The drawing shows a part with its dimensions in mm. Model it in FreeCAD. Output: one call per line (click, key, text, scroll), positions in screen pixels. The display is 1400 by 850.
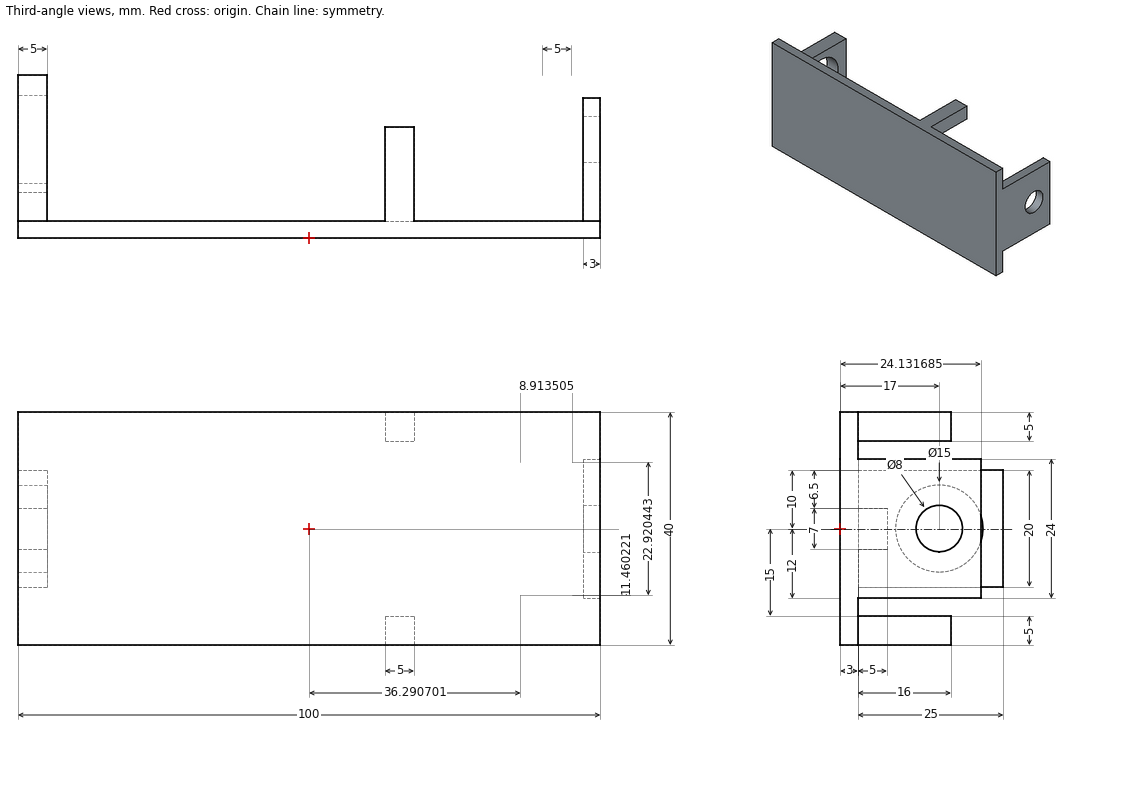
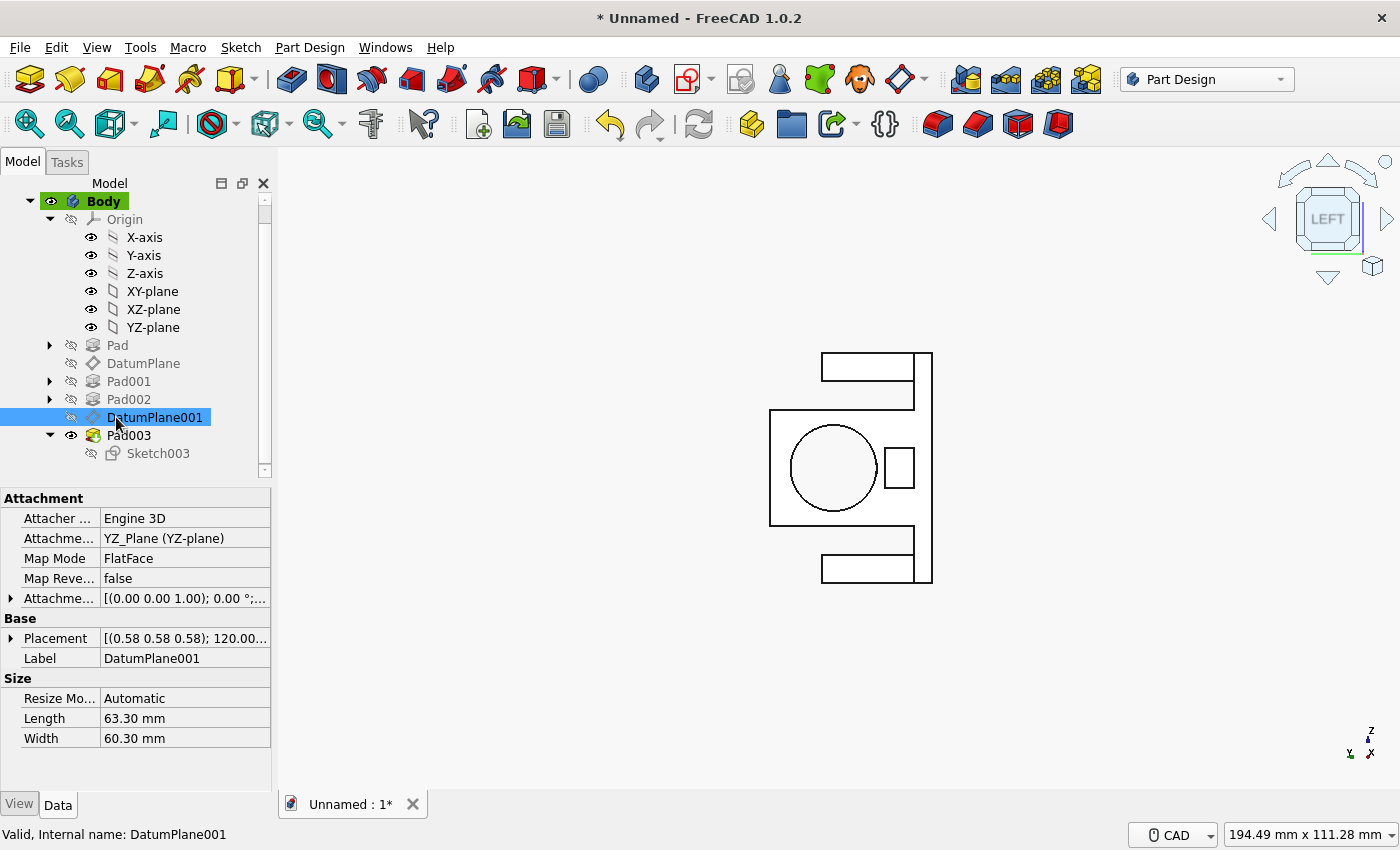
key(v)
key(f)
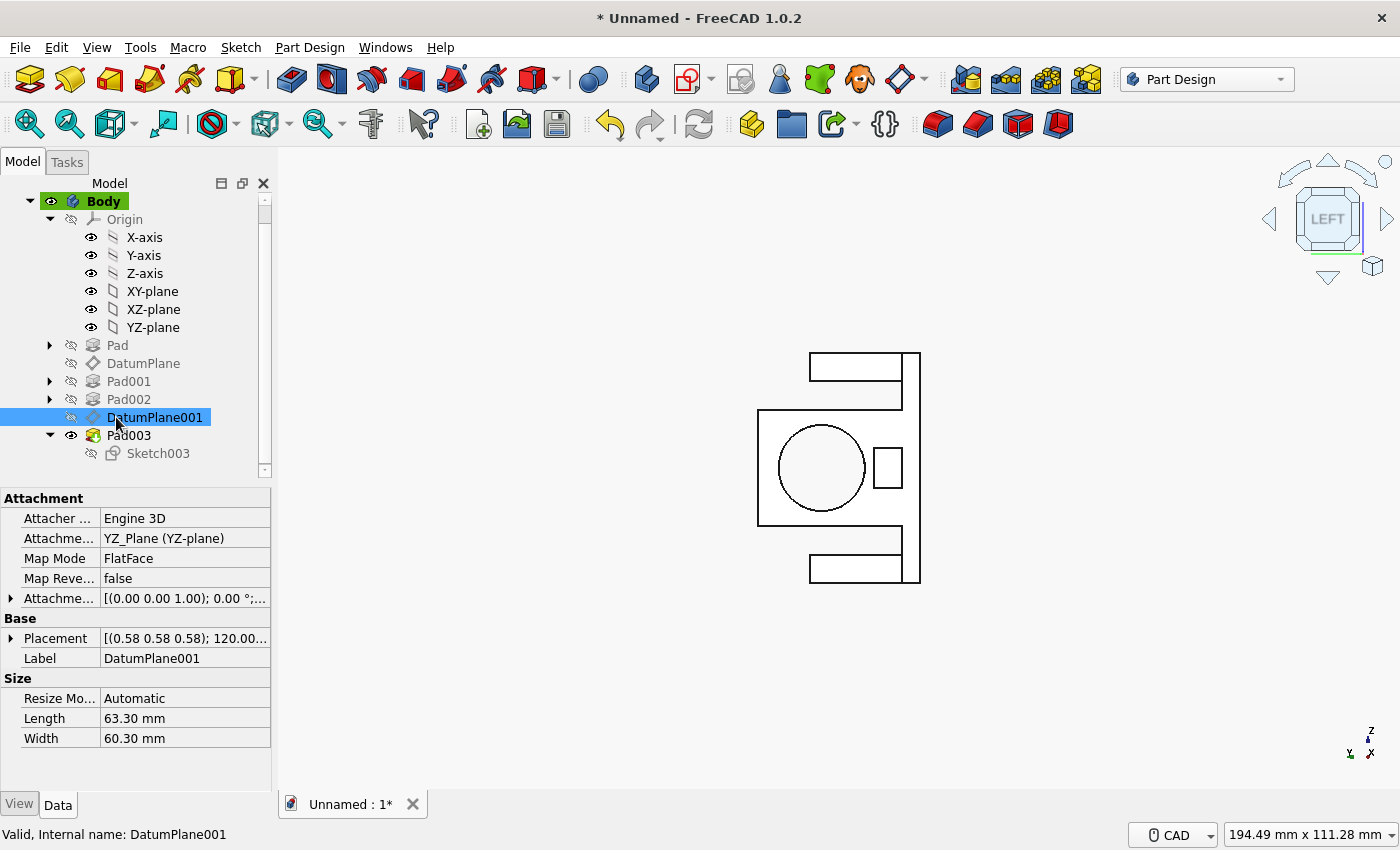
key(0)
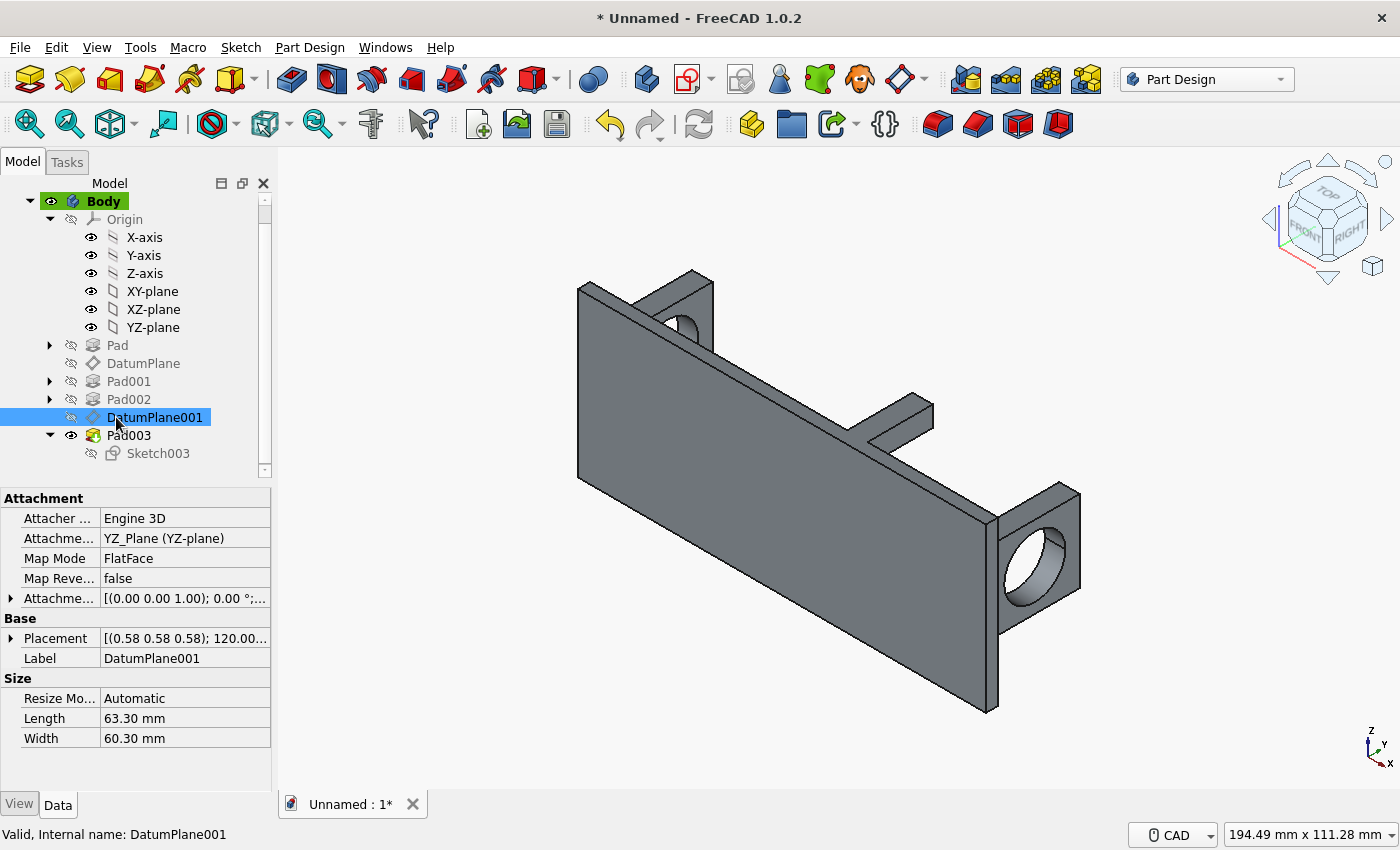
click(994, 532)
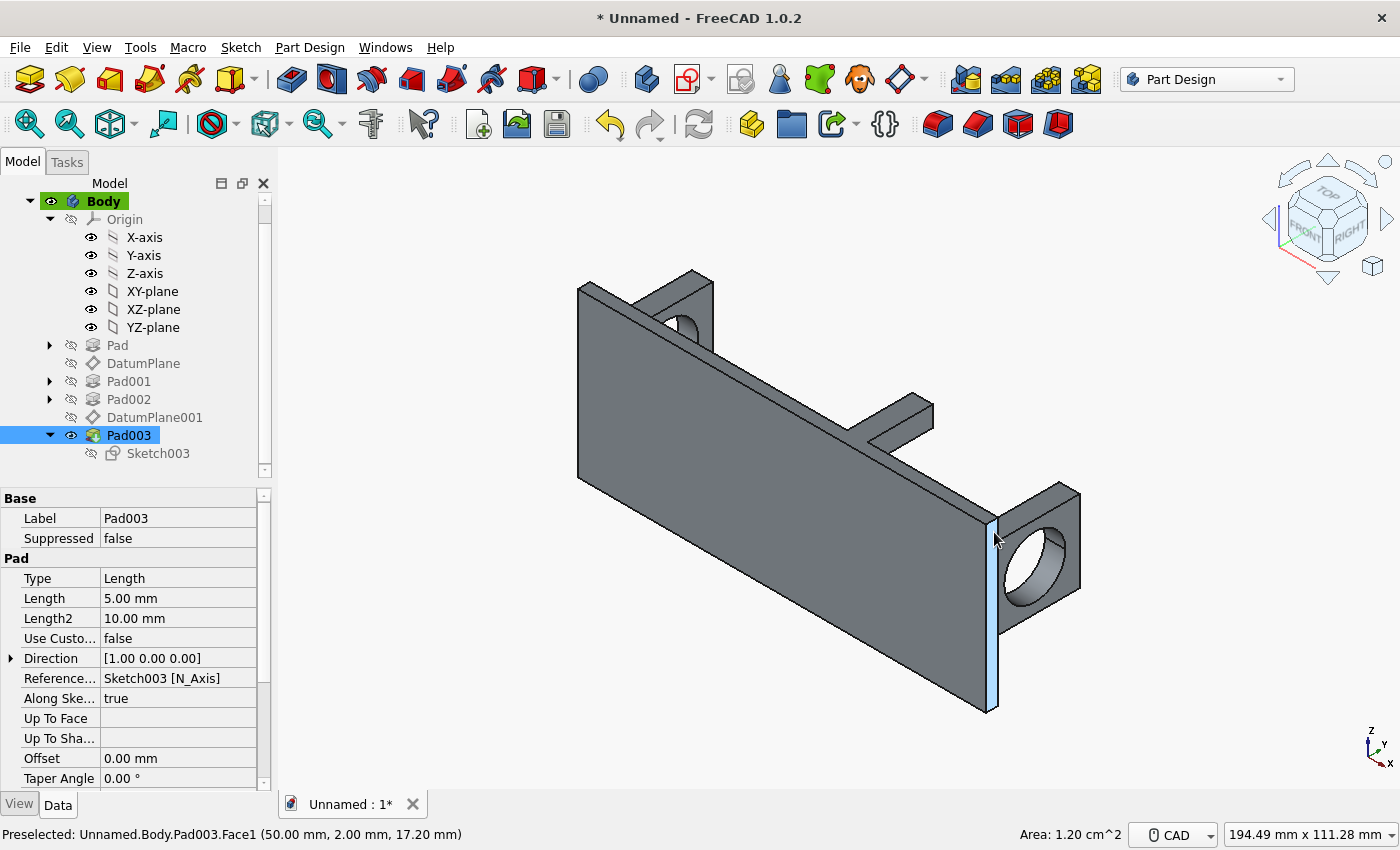
click(688, 80)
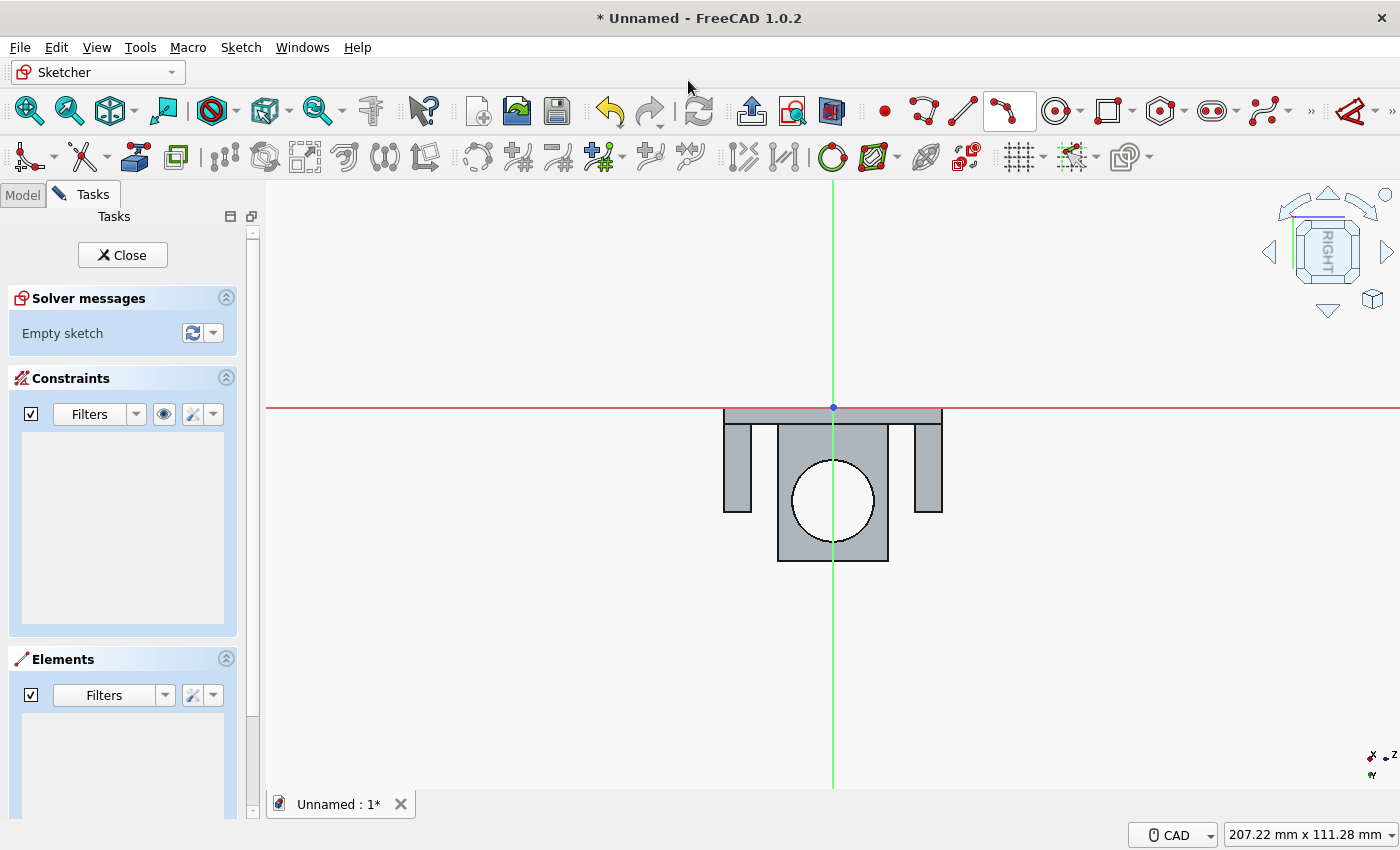
scroll(873, 468, up, 5)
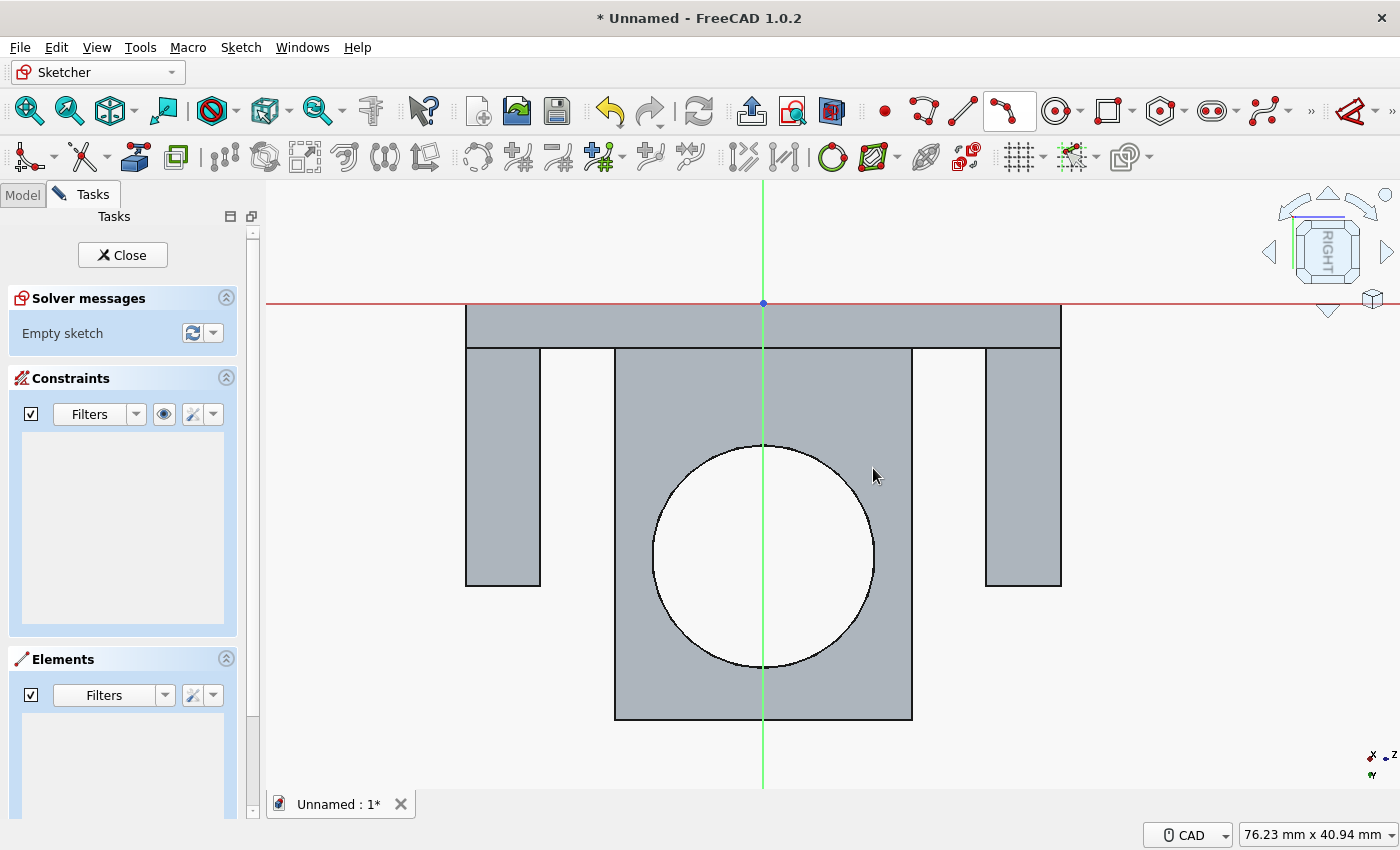
click(1108, 112)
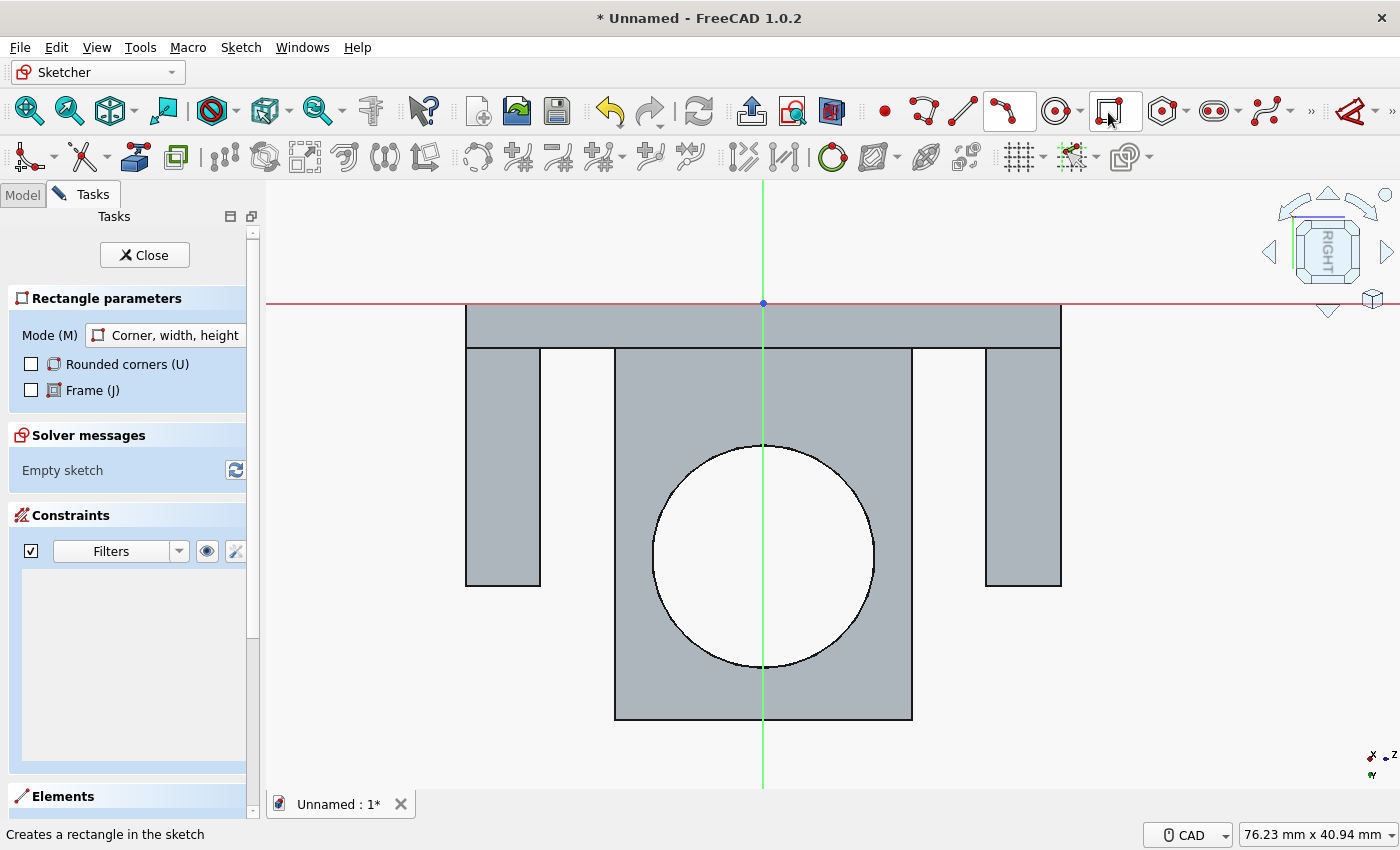
click(585, 304)
move(942, 663)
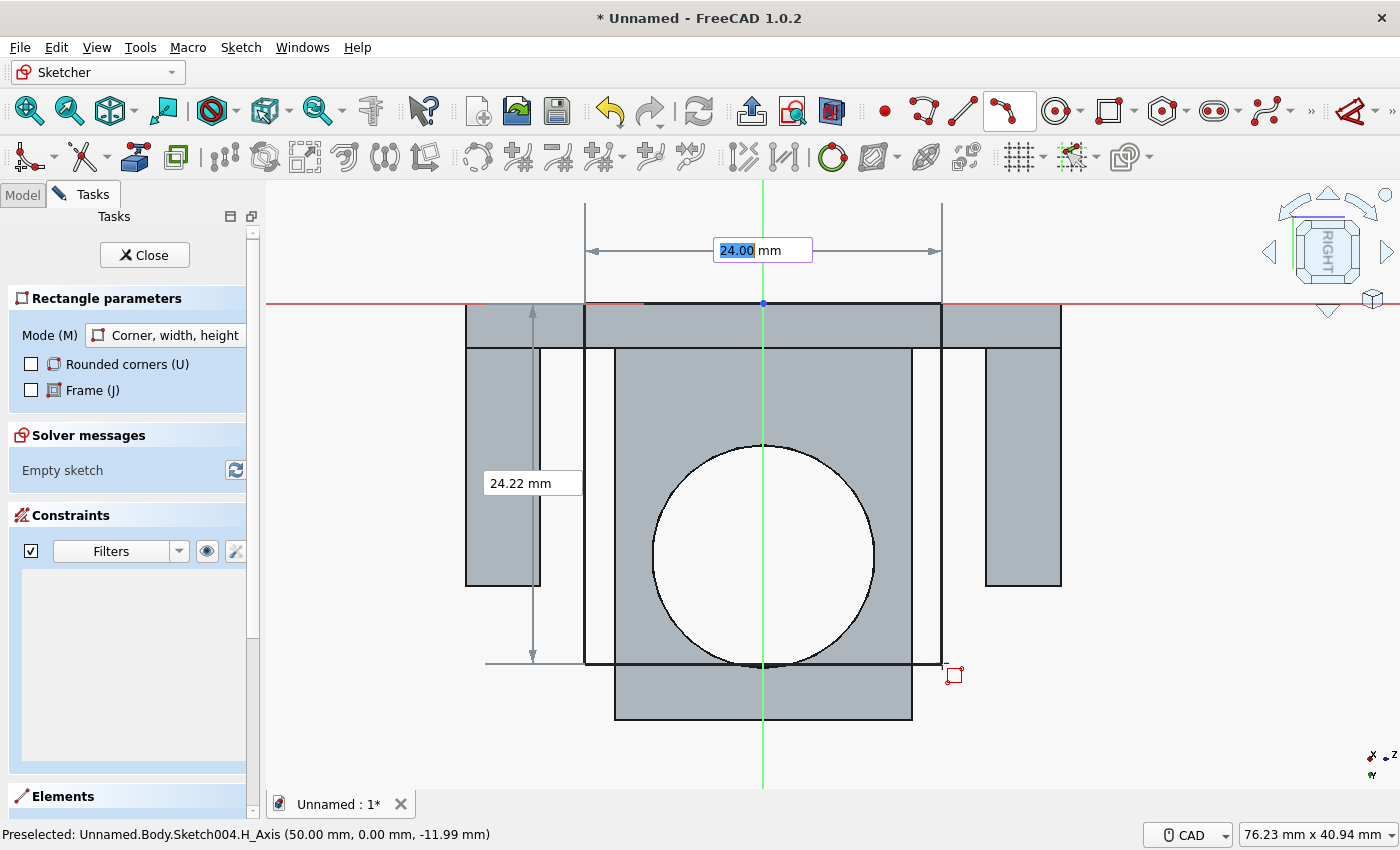
text(24)
key(Tab)
text(24.131685)
key(Return)